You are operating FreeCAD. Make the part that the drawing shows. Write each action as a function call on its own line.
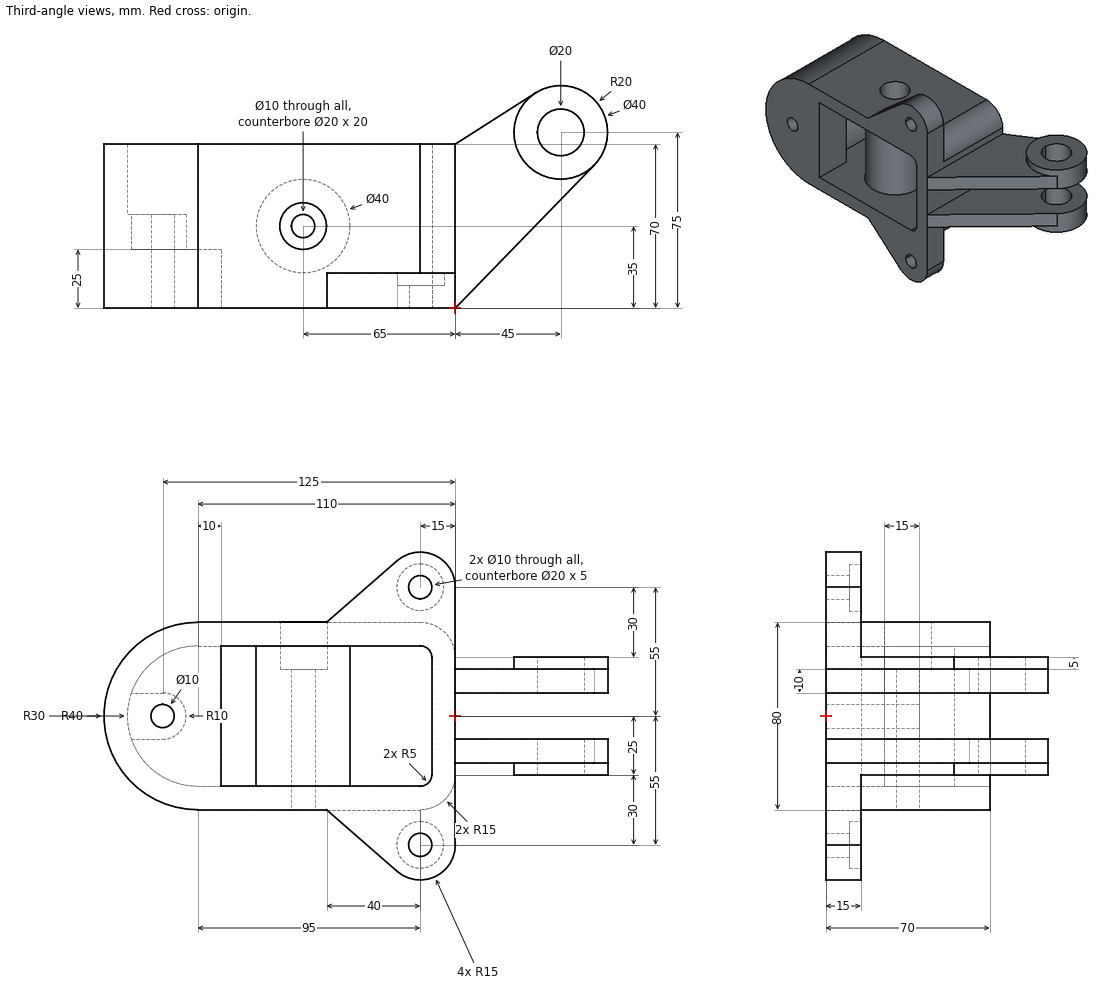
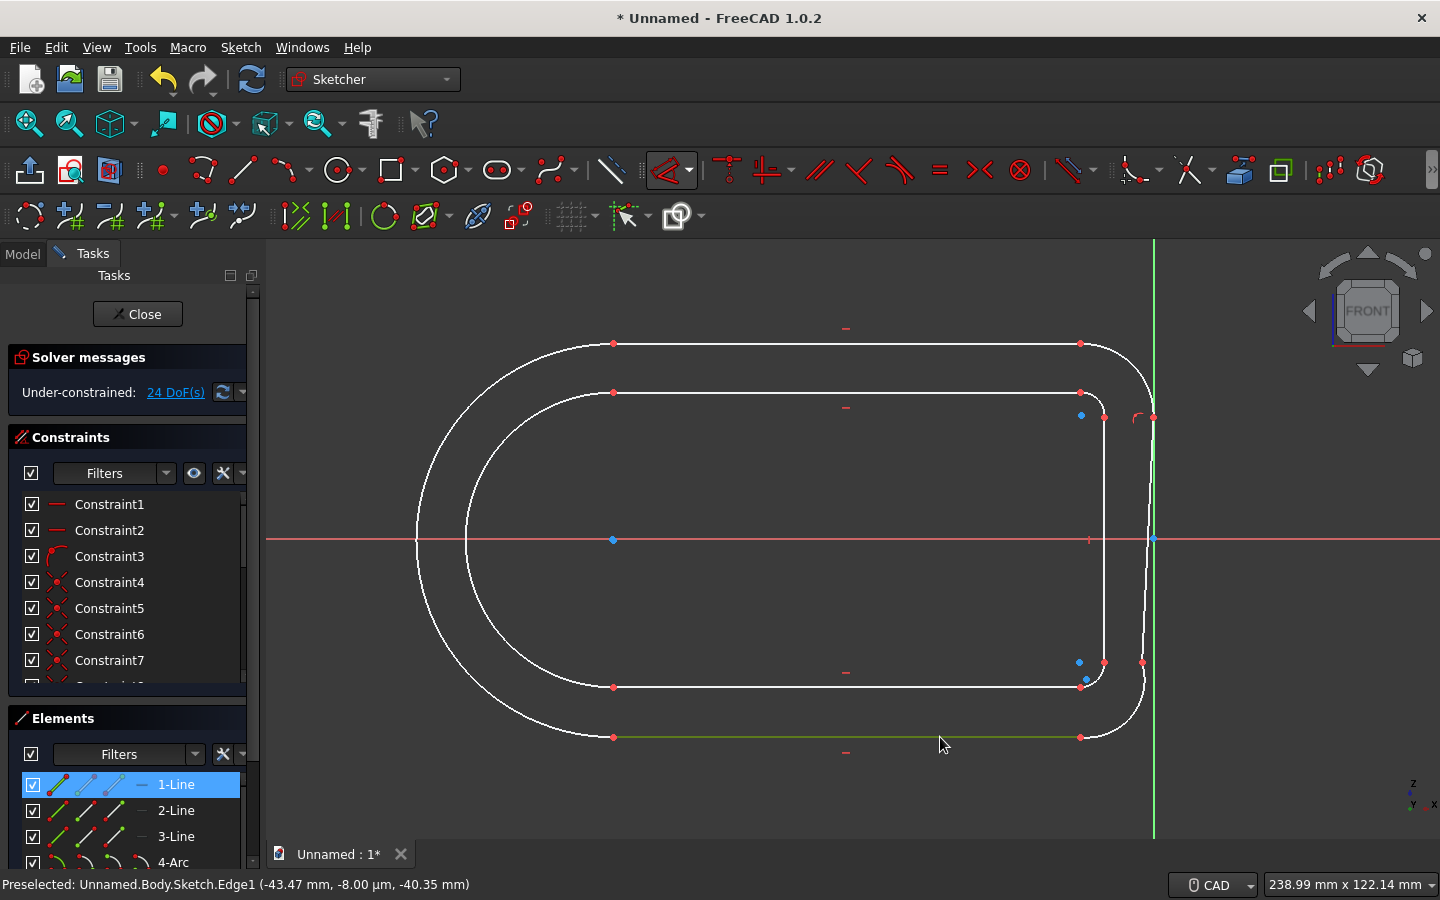
click(1113, 731)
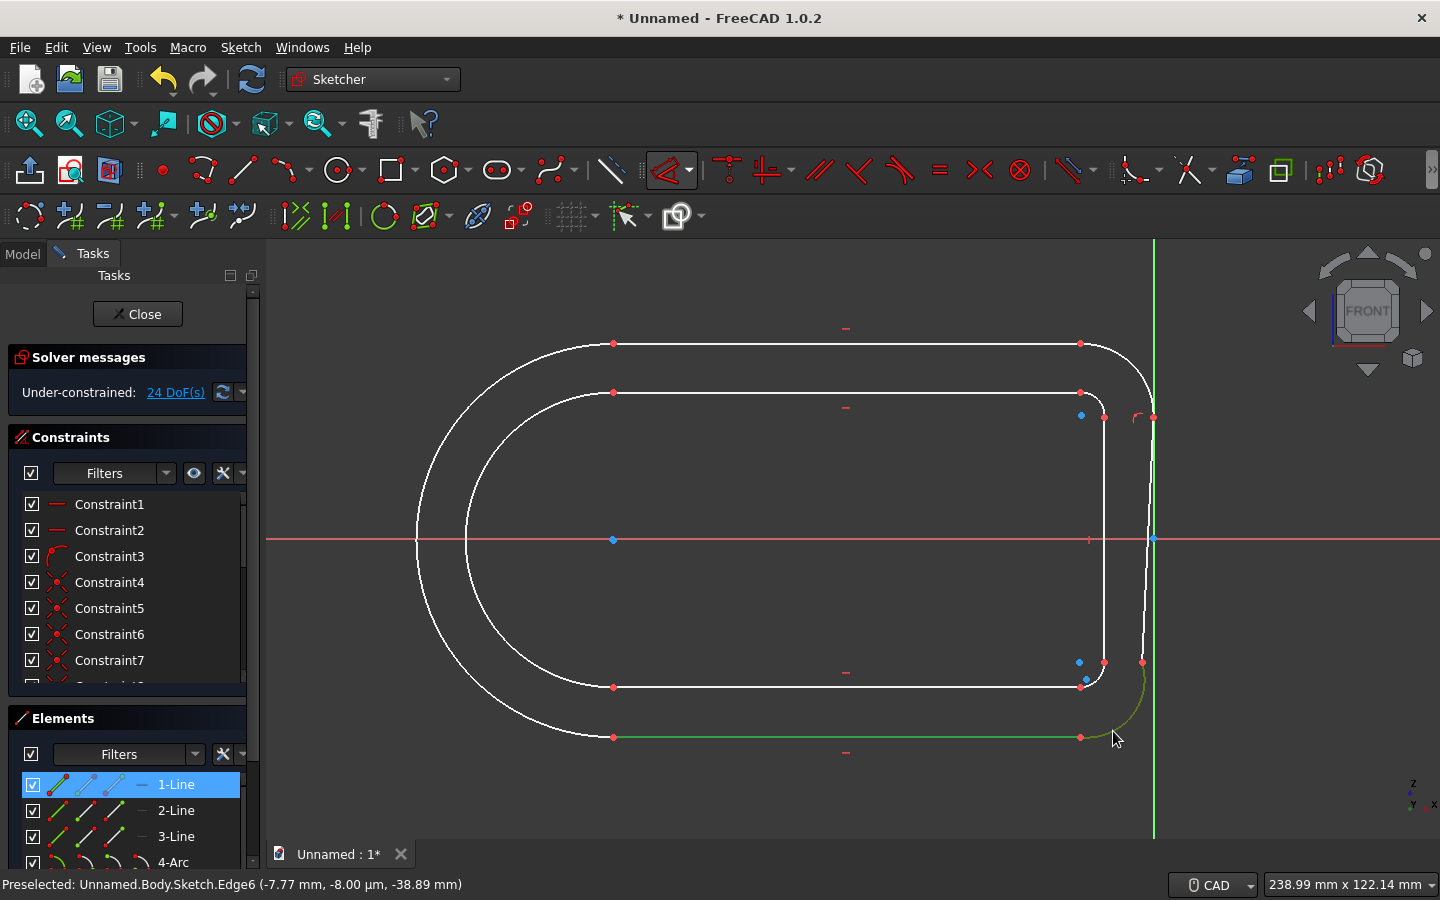
click(900, 170)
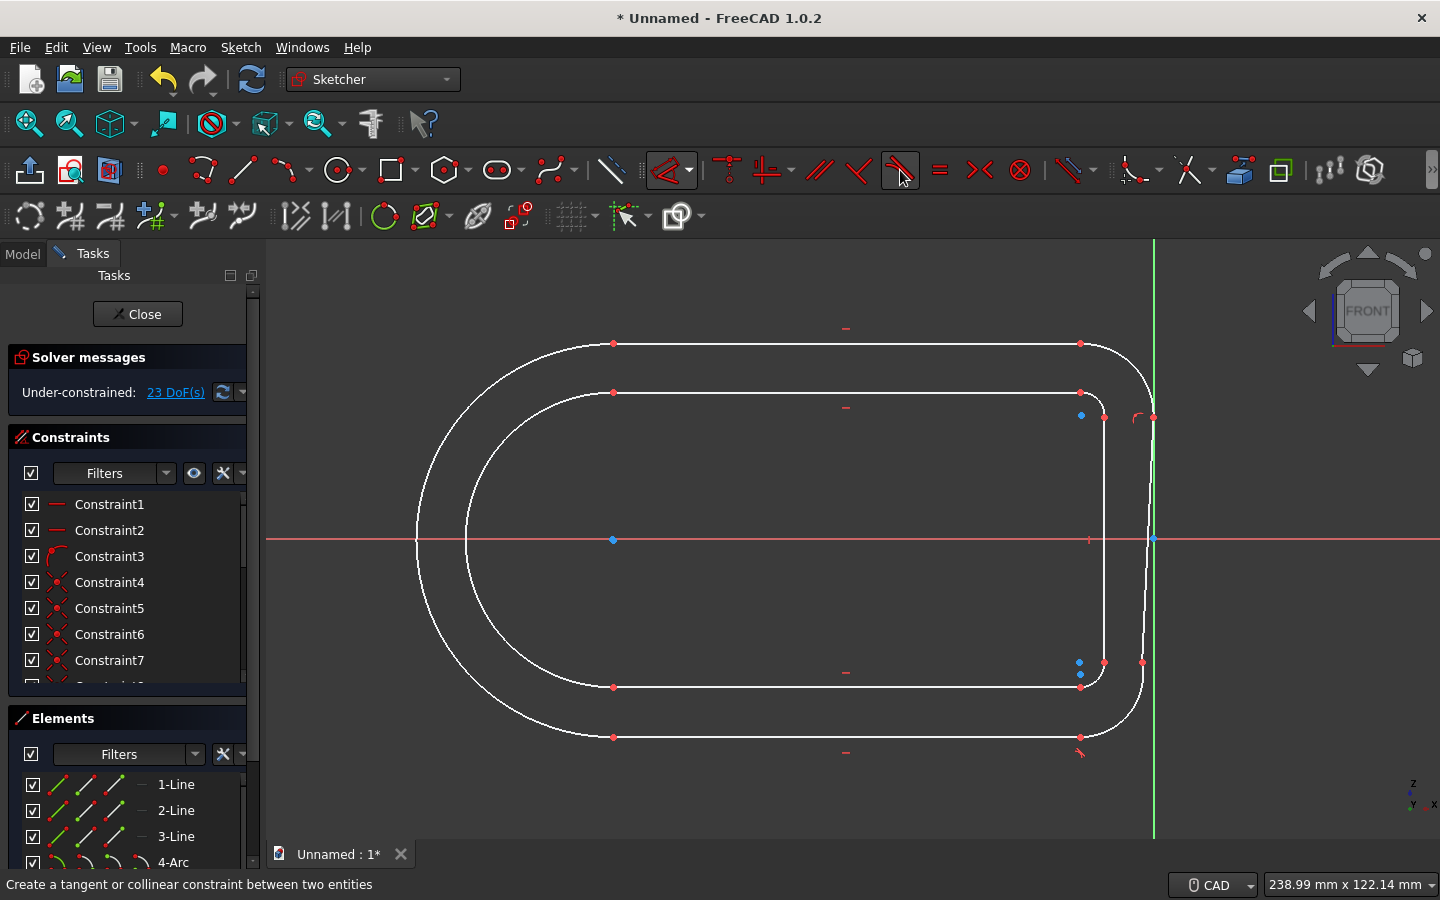
click(754, 344)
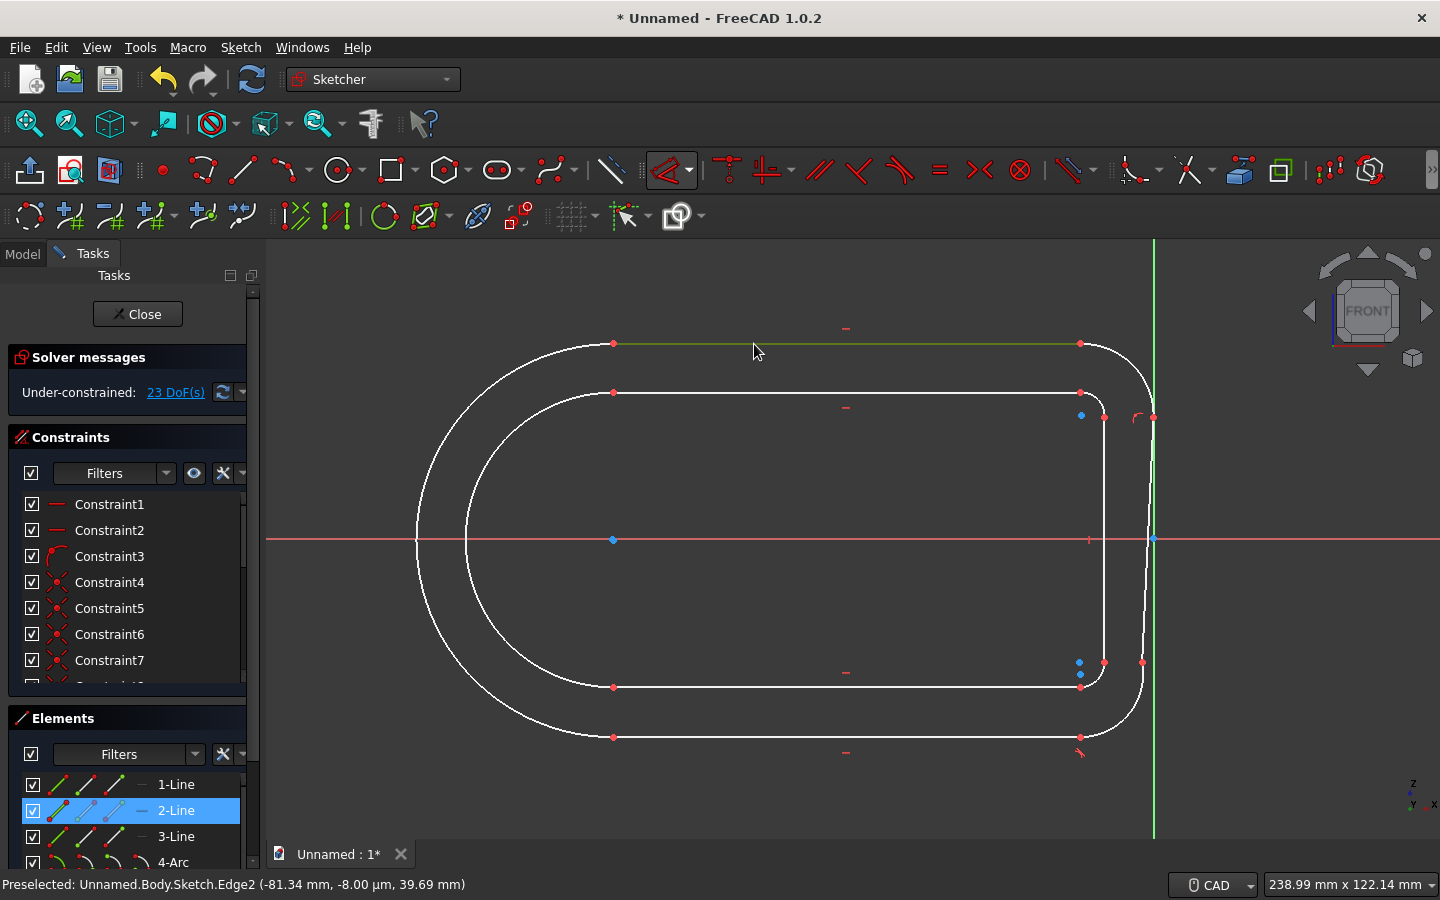
click(1114, 351)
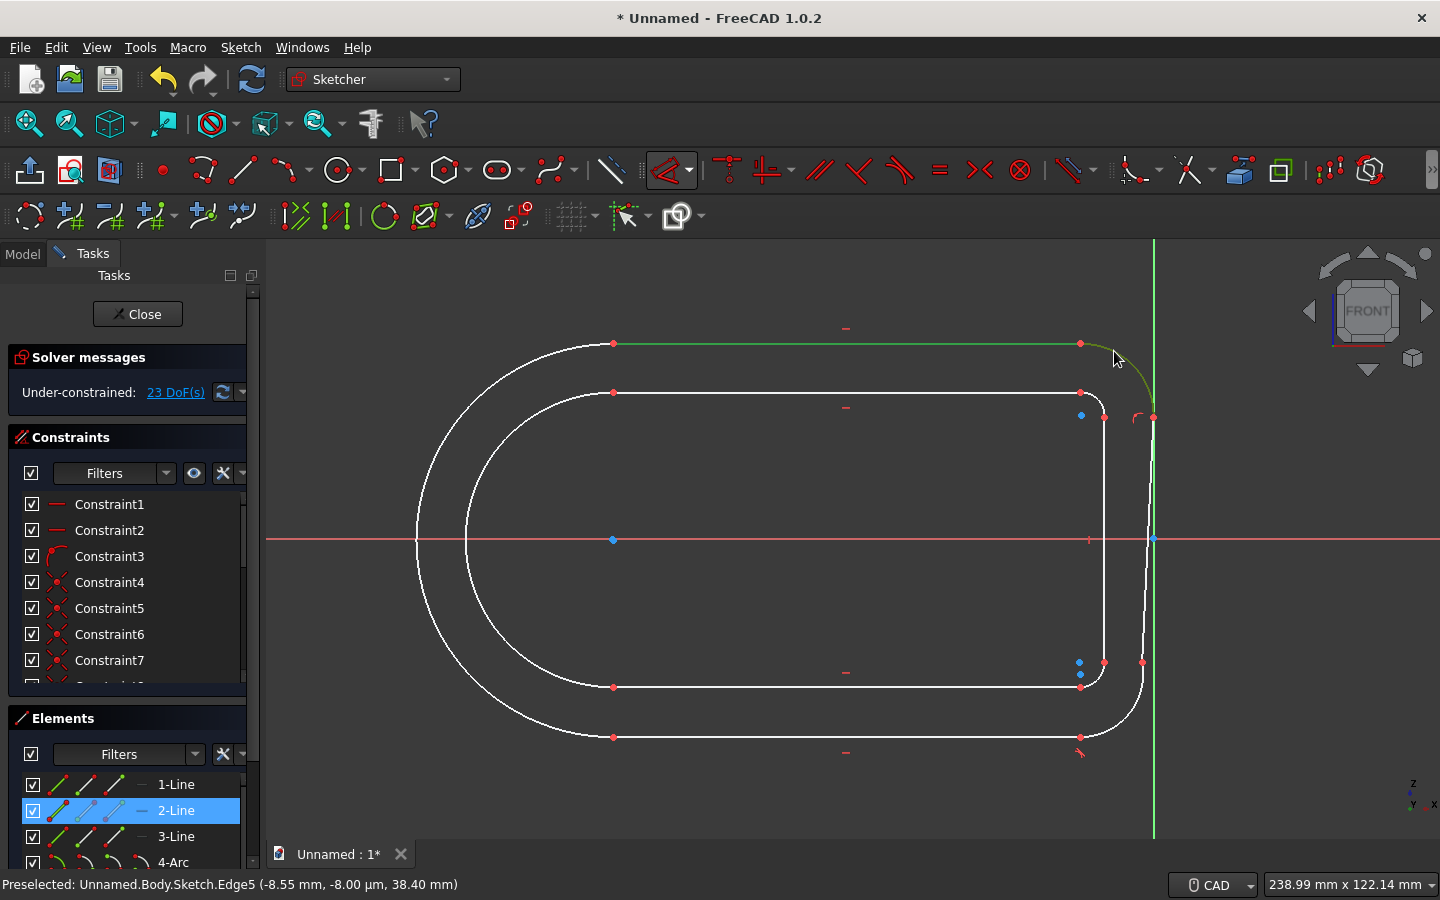
click(900, 170)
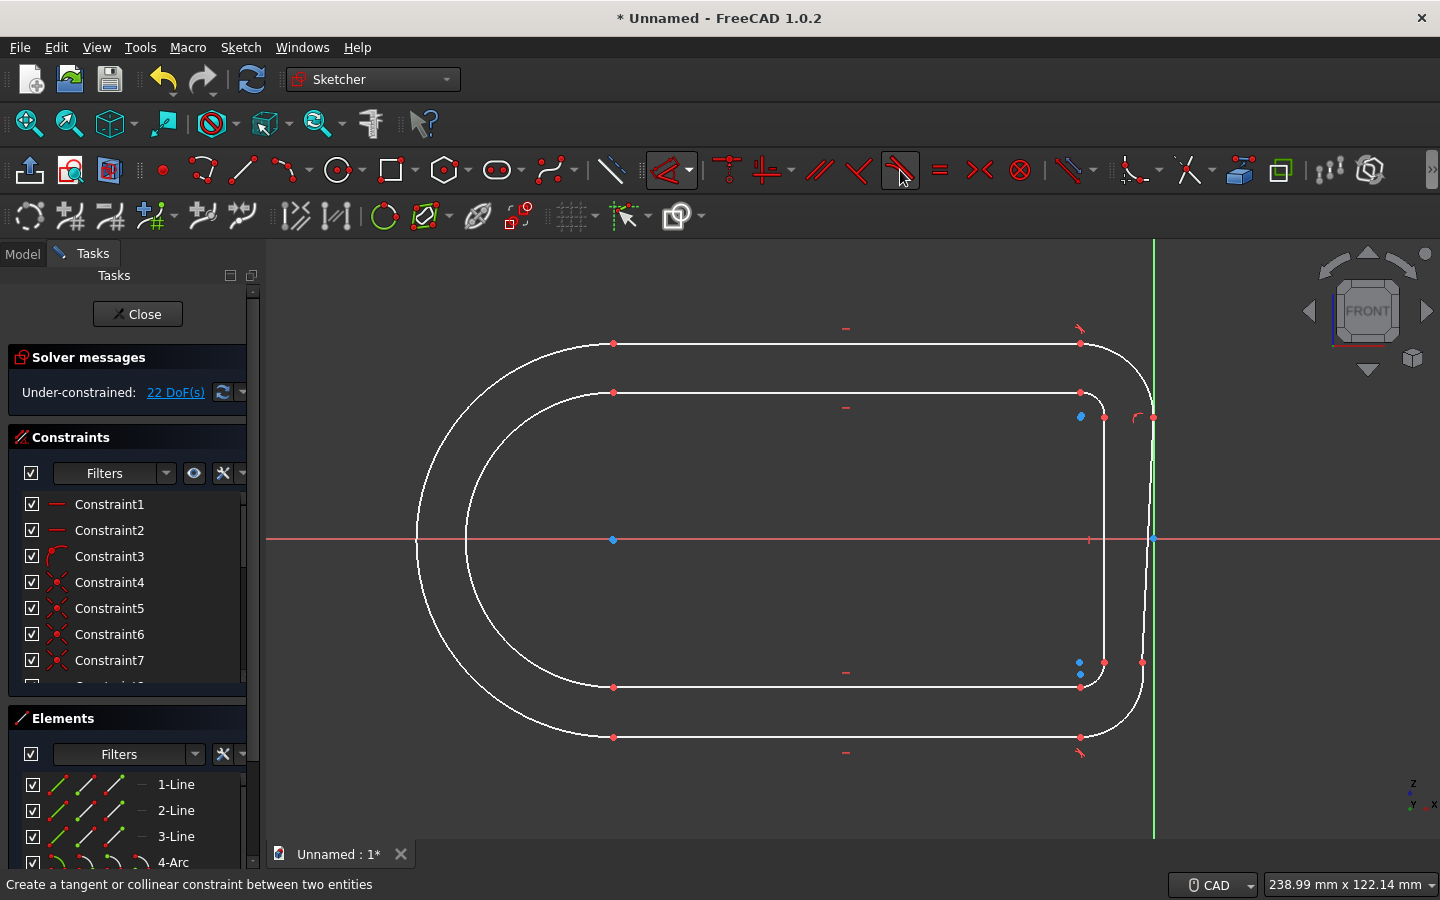
click(1150, 491)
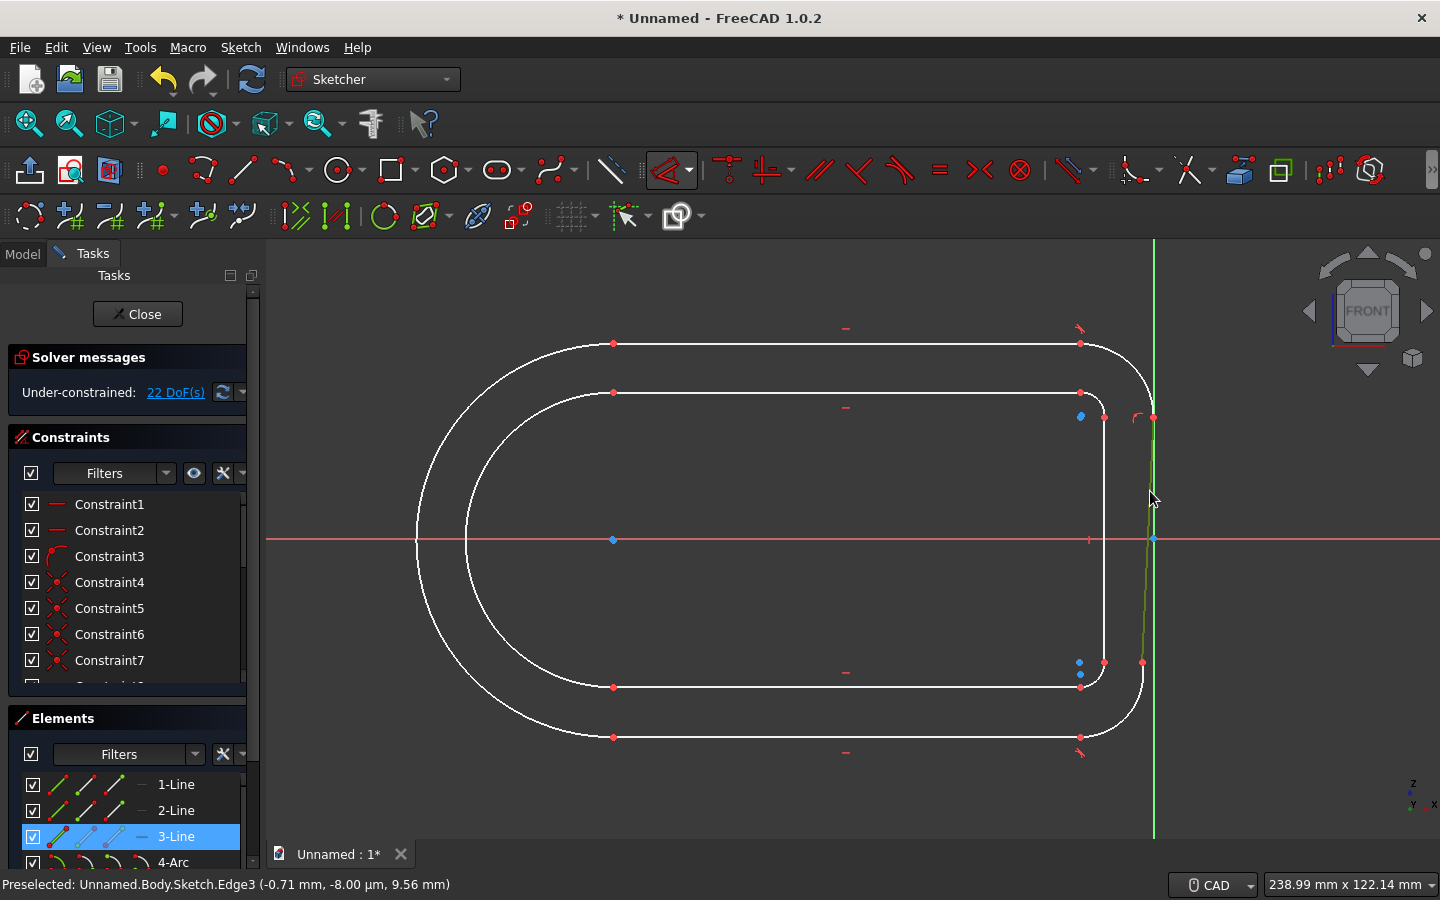
click(1113, 352)